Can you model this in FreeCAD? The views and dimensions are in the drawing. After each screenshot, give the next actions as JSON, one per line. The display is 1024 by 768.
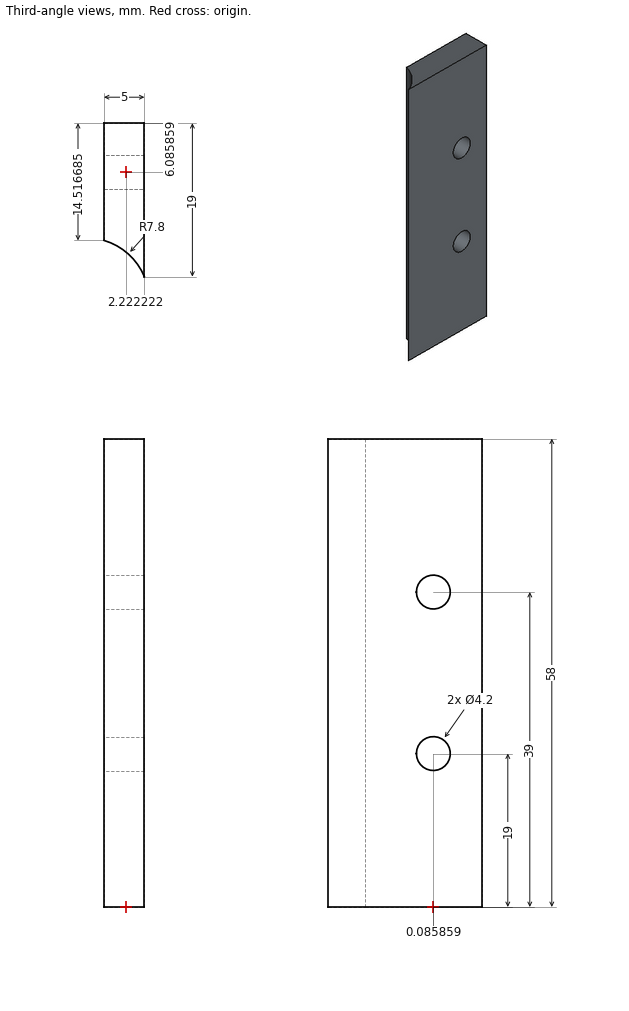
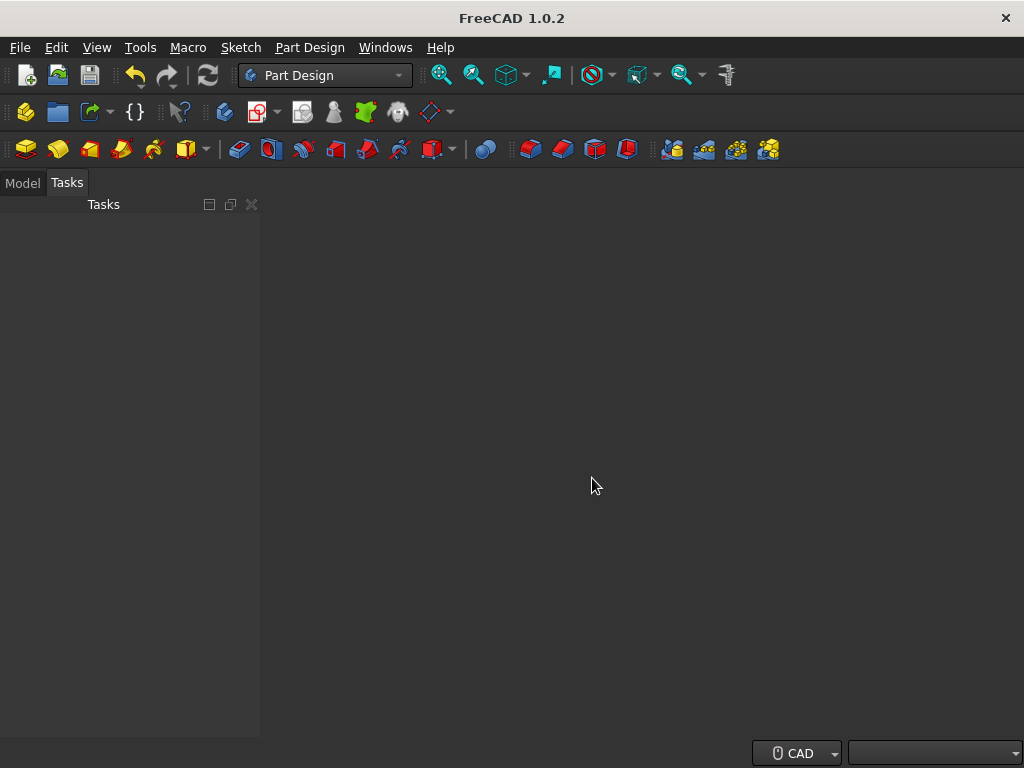
{"action": "left_click", "coordinate": [26, 76]}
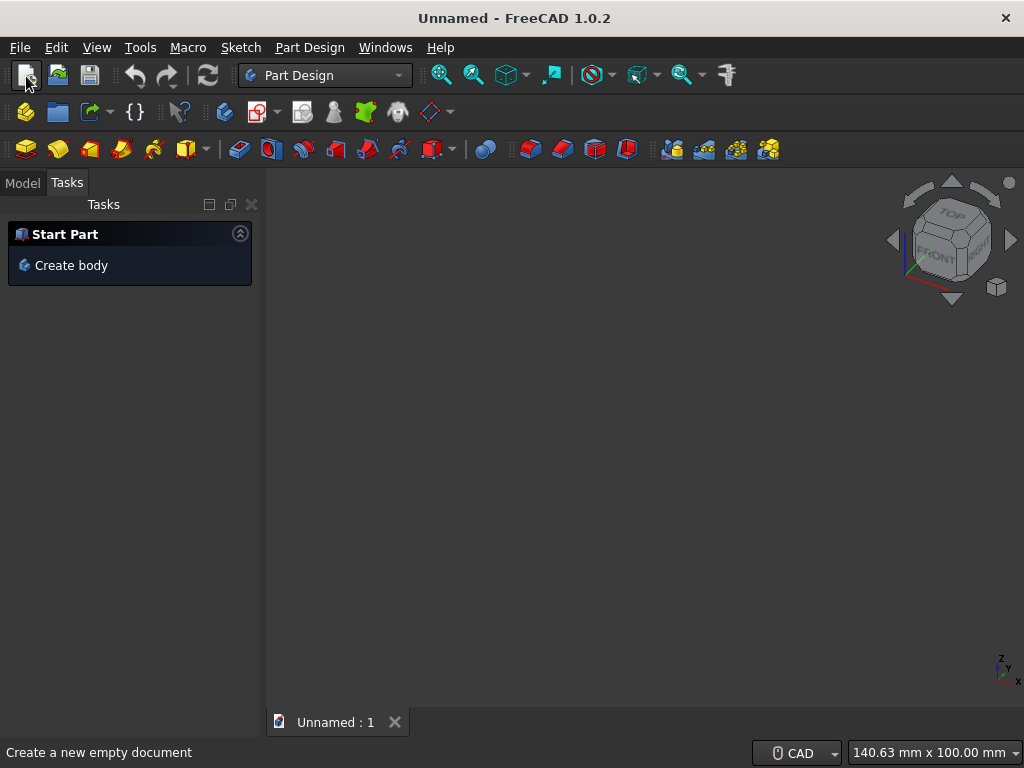
{"action": "left_click", "coordinate": [258, 112]}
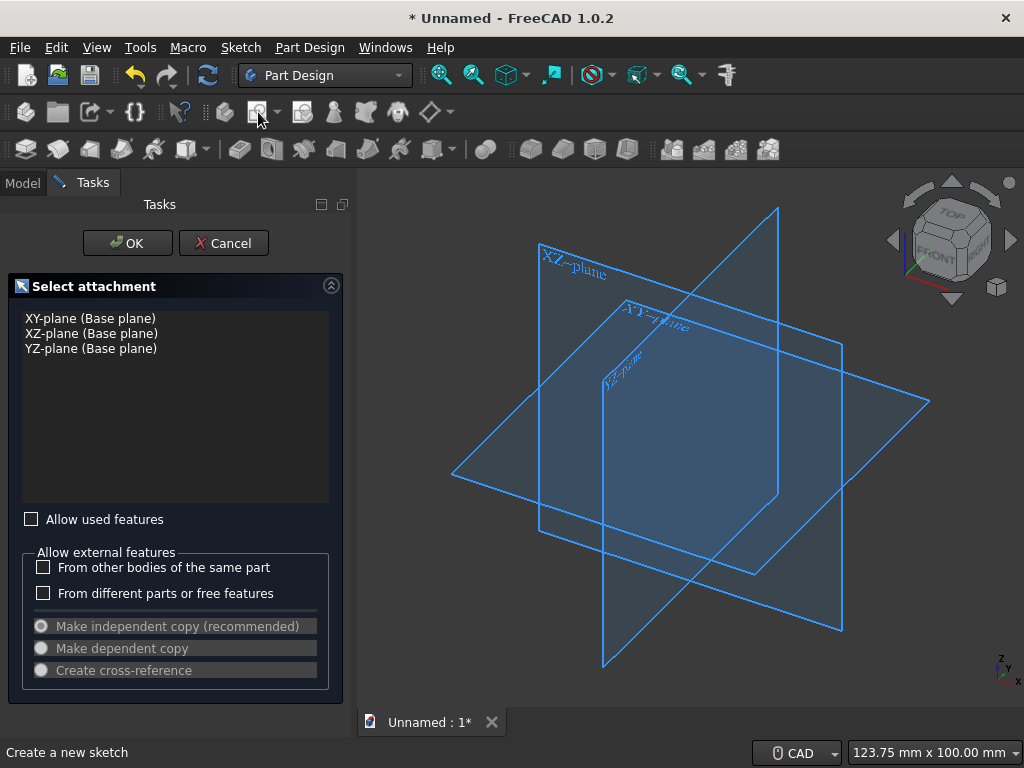
{"action": "left_click", "coordinate": [82, 318]}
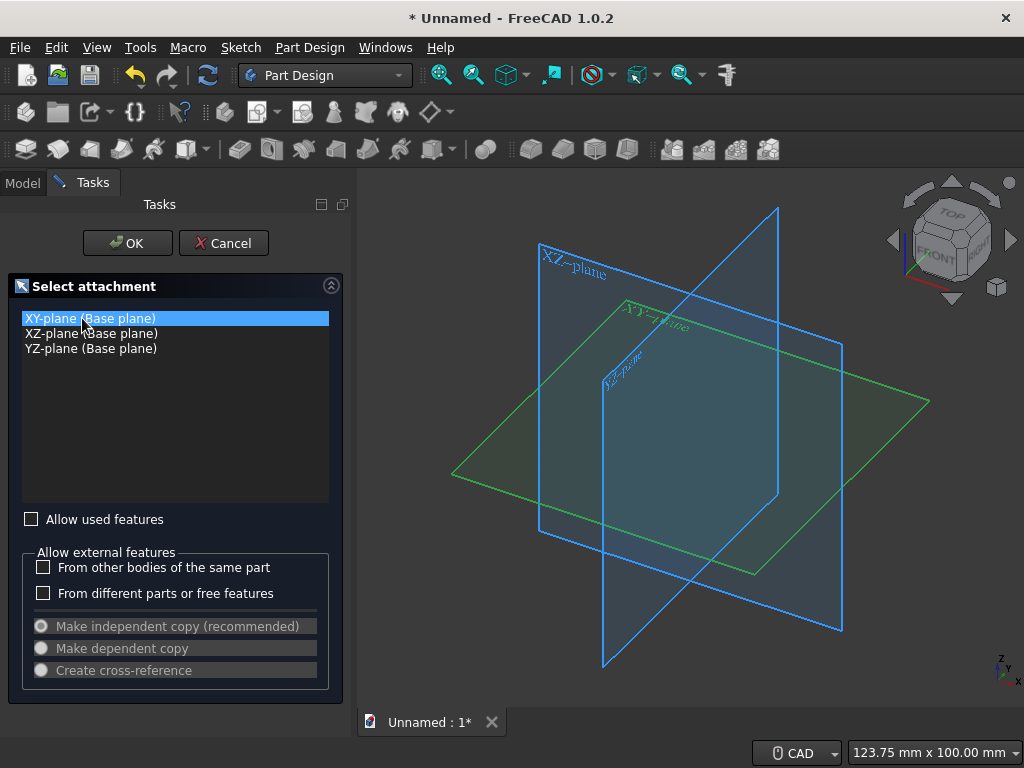
{"action": "left_click", "coordinate": [128, 243]}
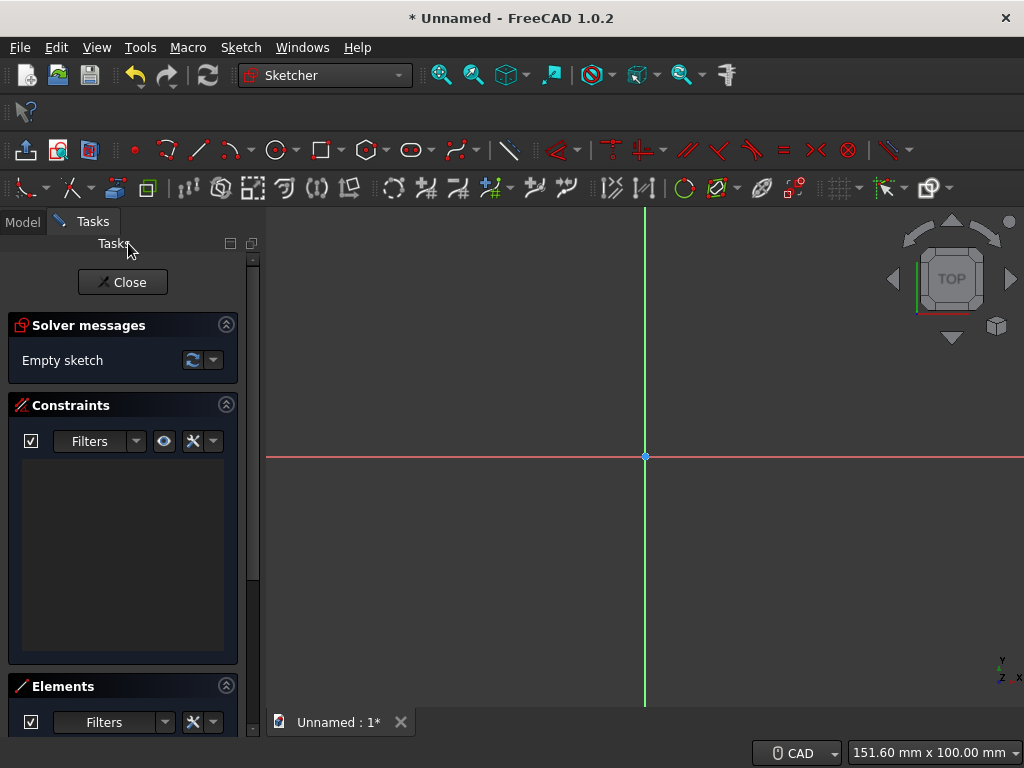
{"action": "scroll", "coordinate": [673, 481], "scroll_direction": "up", "scroll_amount": 6}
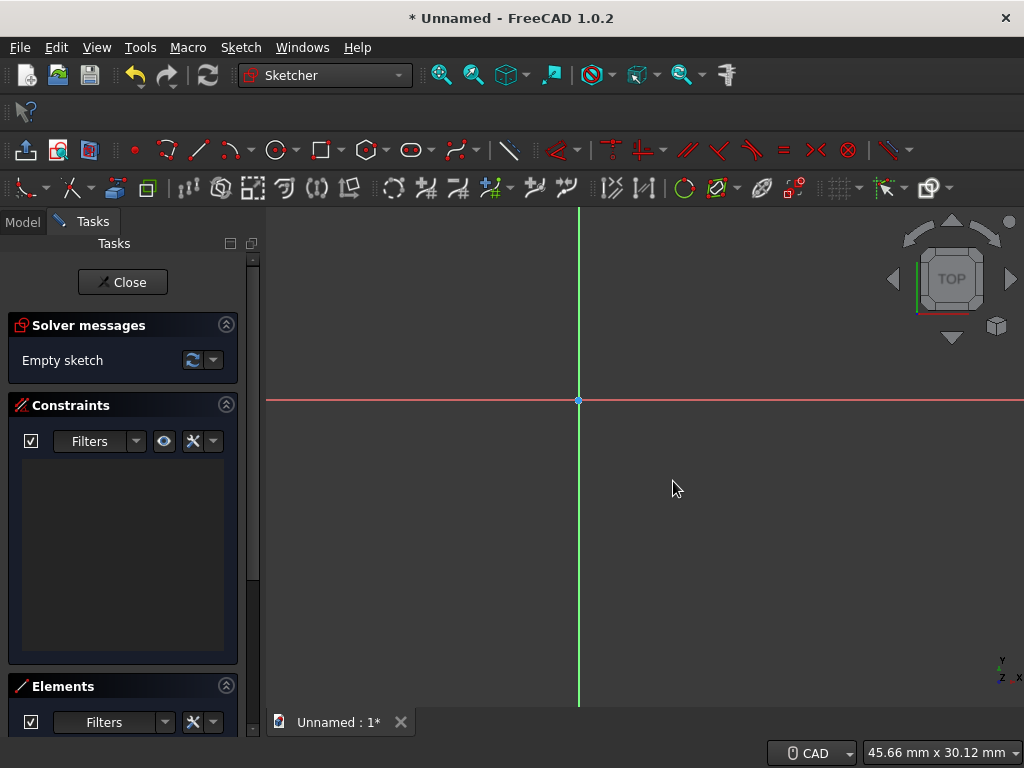
{"action": "left_click", "coordinate": [168, 150]}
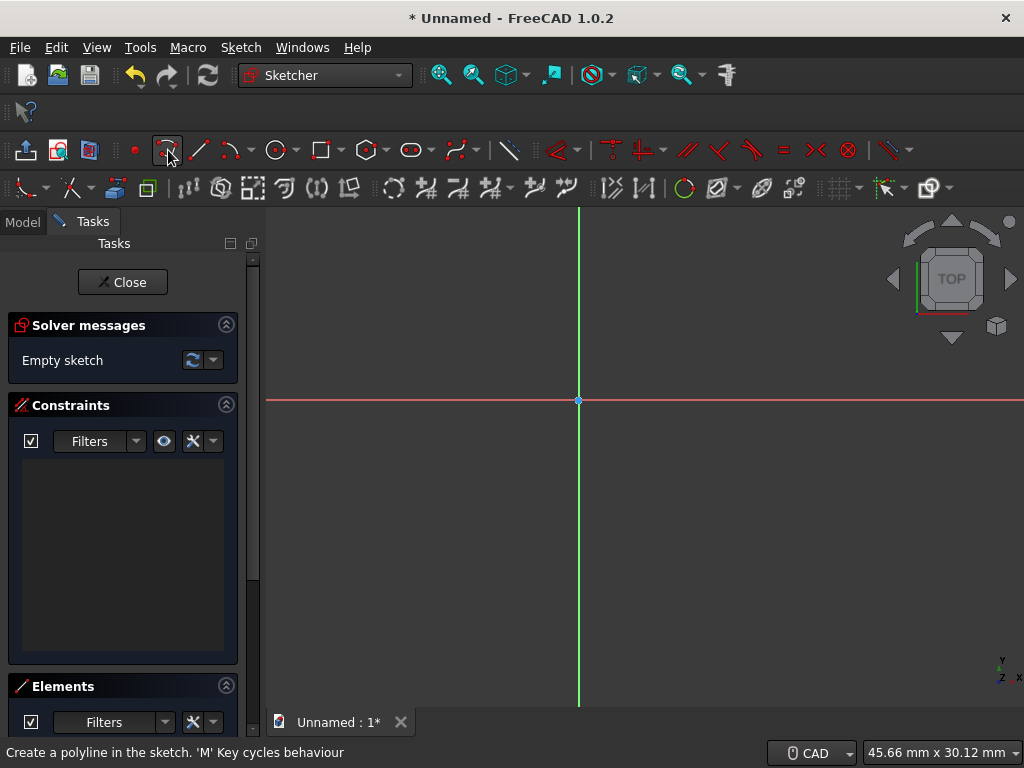
{"action": "left_click", "coordinate": [616, 614]}
{"action": "left_click", "coordinate": [616, 299]}
{"action": "left_click", "coordinate": [533, 299]}
{"action": "left_click", "coordinate": [533, 540]}
{"action": "right_click", "coordinate": [533, 540]}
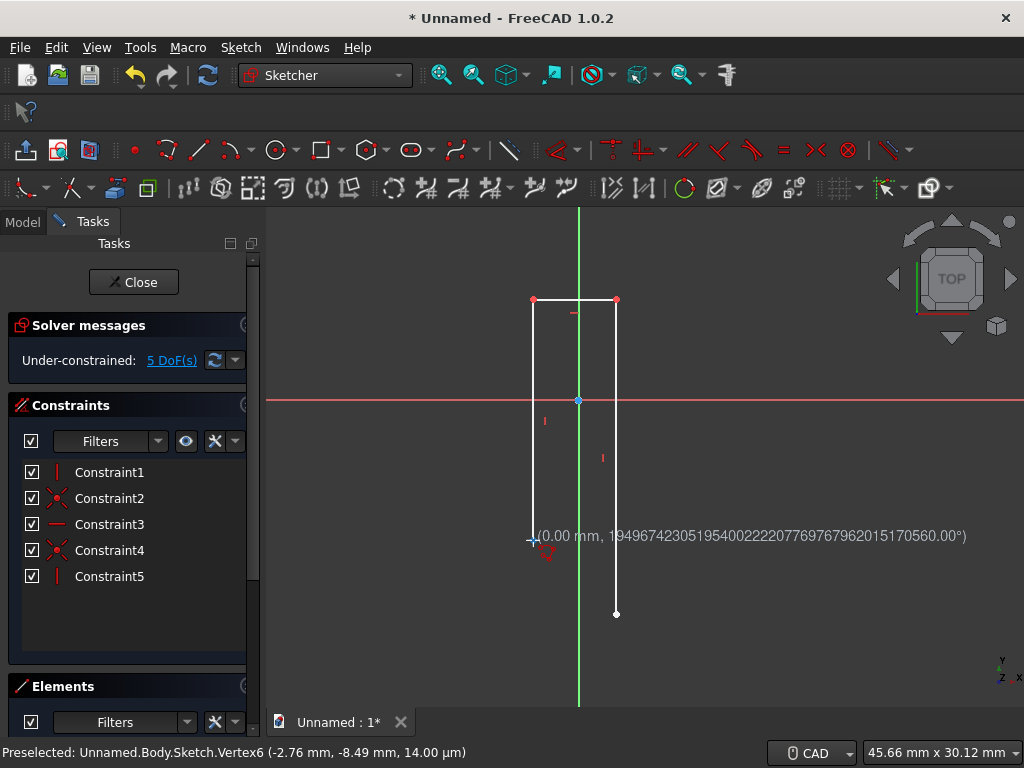
{"action": "left_click", "coordinate": [254, 150]}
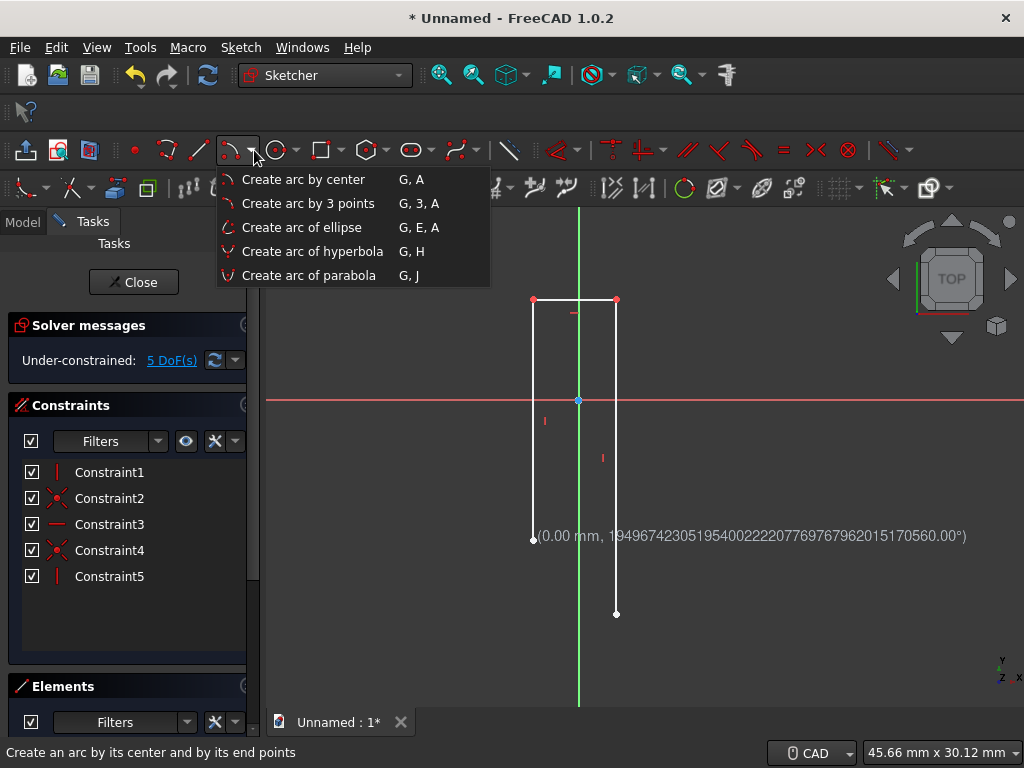
{"action": "left_click", "coordinate": [354, 203]}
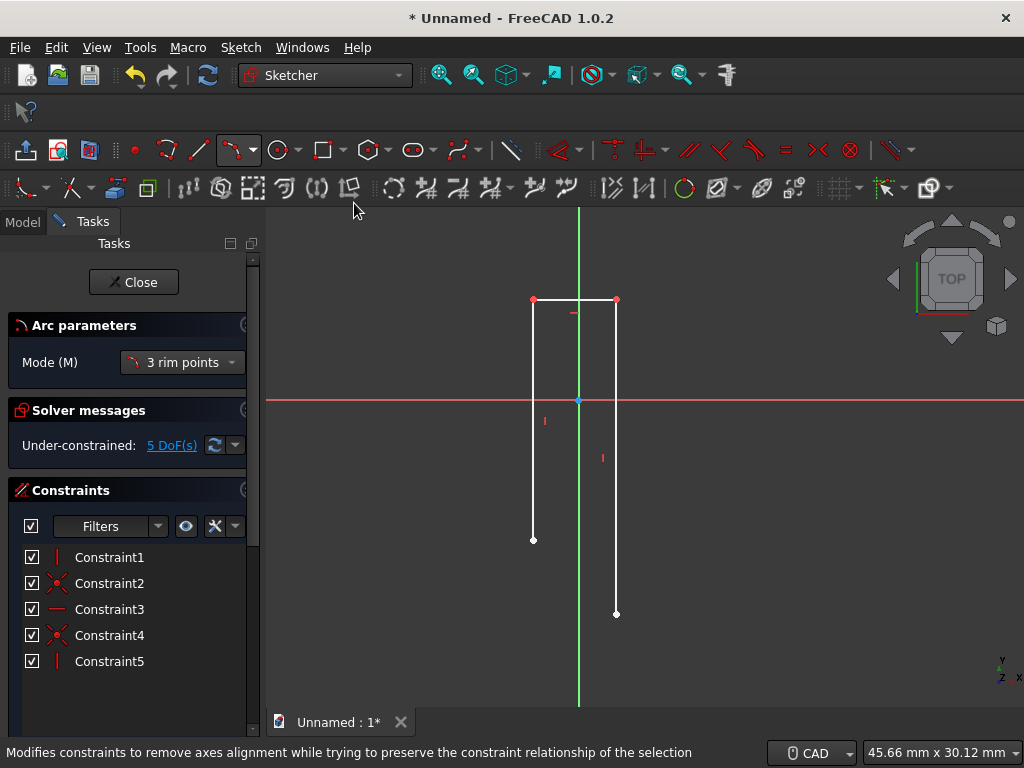
{"action": "left_click", "coordinate": [533, 541]}
{"action": "left_click", "coordinate": [616, 615]}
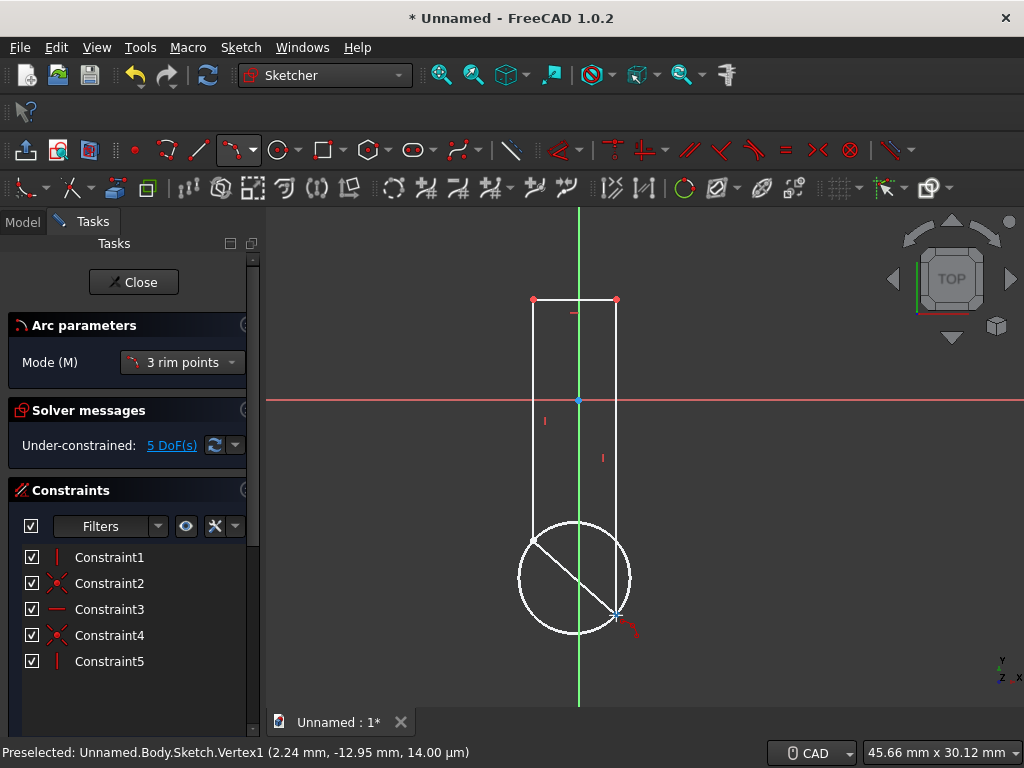
{"action": "scroll", "coordinate": [591, 576], "scroll_direction": "up", "scroll_amount": 2}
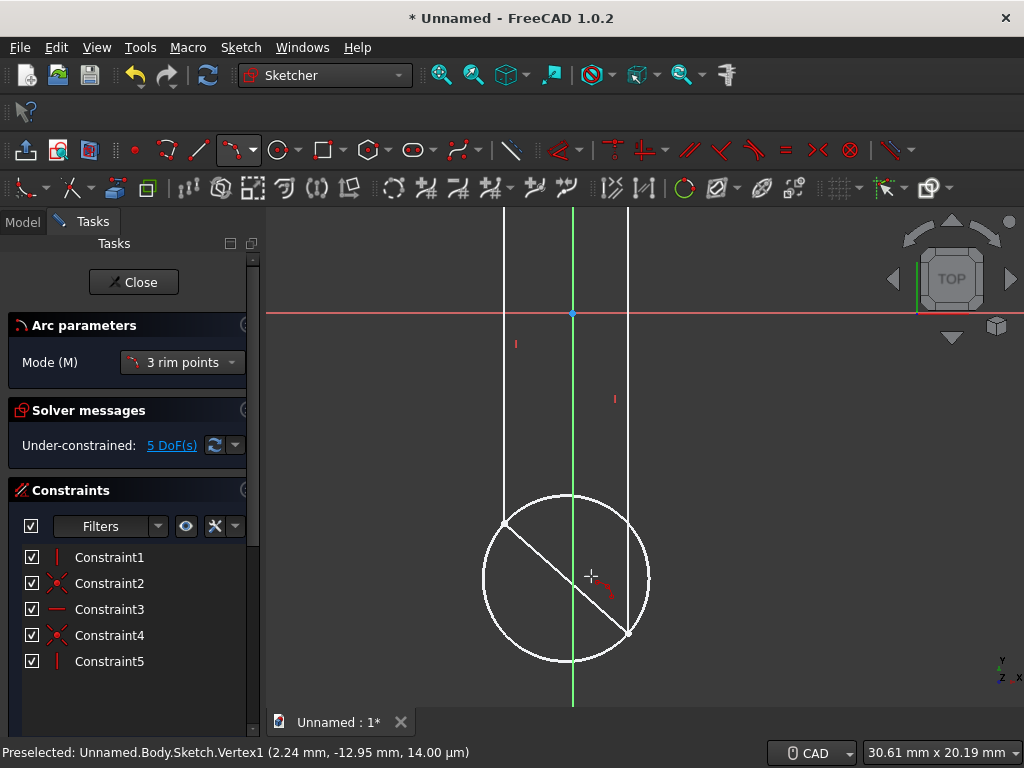
{"action": "left_click", "coordinate": [591, 575]}
{"action": "key", "text": "Escape"}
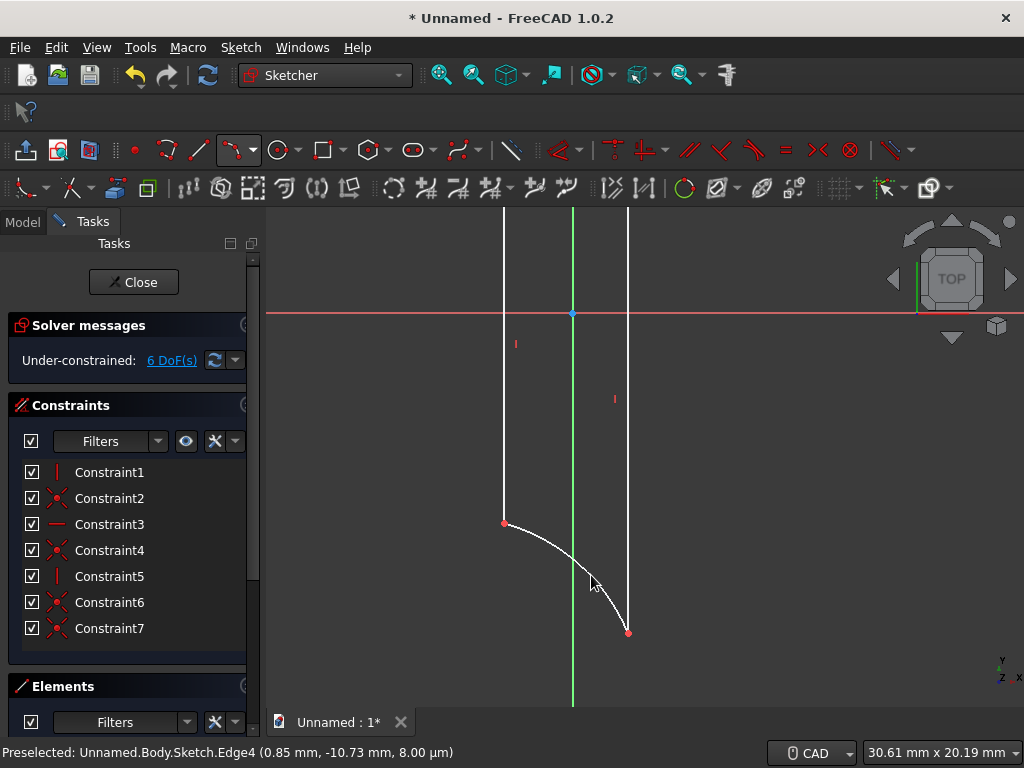
{"action": "left_click", "coordinate": [558, 150]}